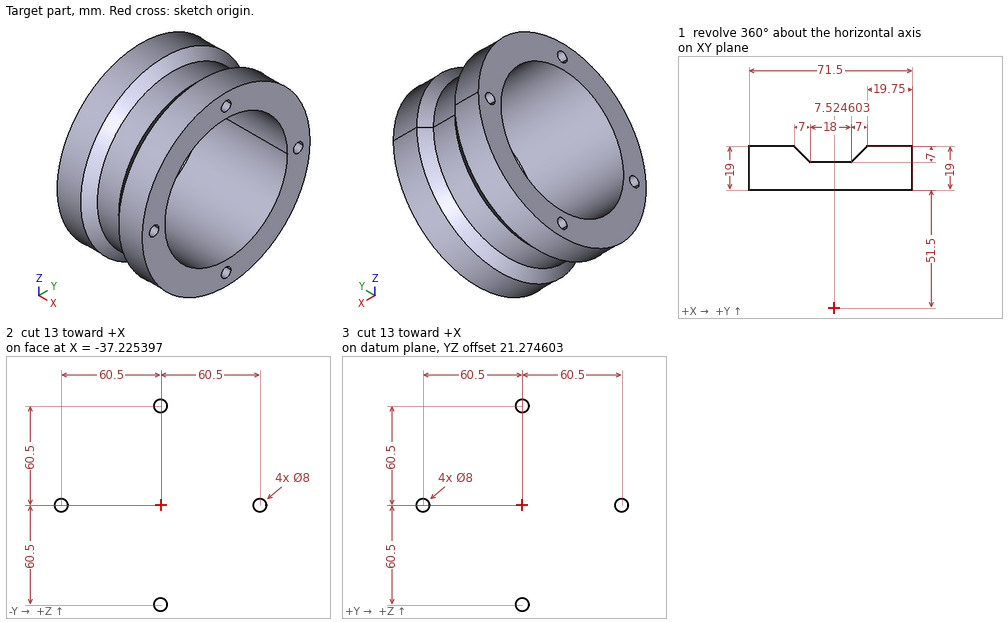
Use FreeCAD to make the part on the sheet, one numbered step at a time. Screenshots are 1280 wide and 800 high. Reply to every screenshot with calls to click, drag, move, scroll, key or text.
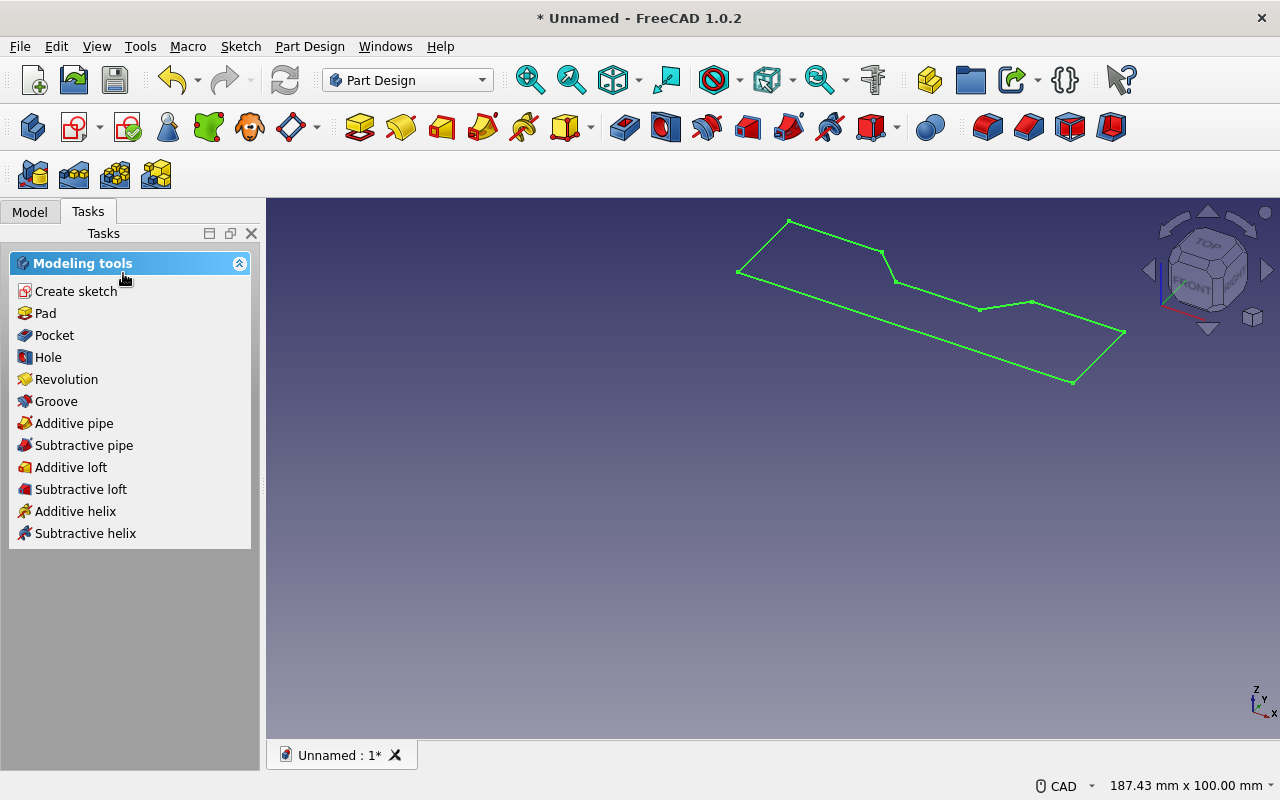
click(401, 128)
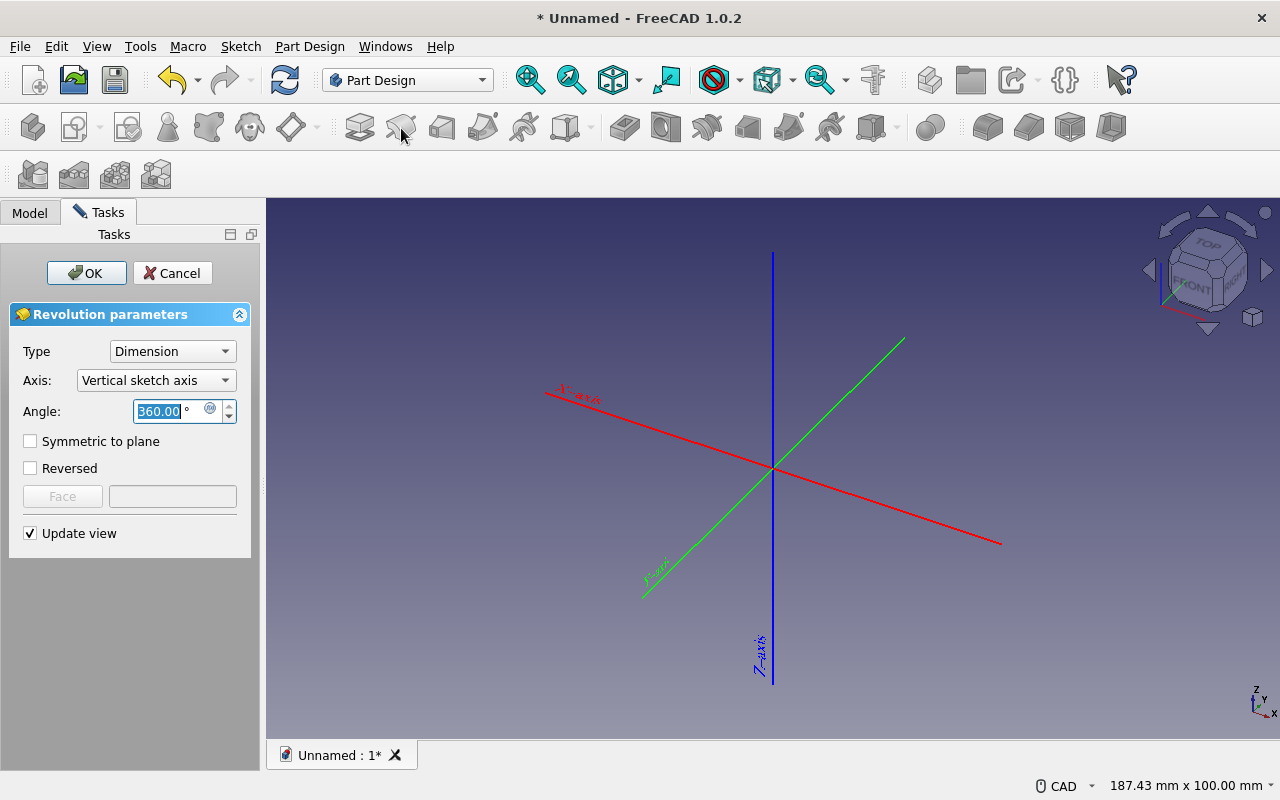
click(157, 380)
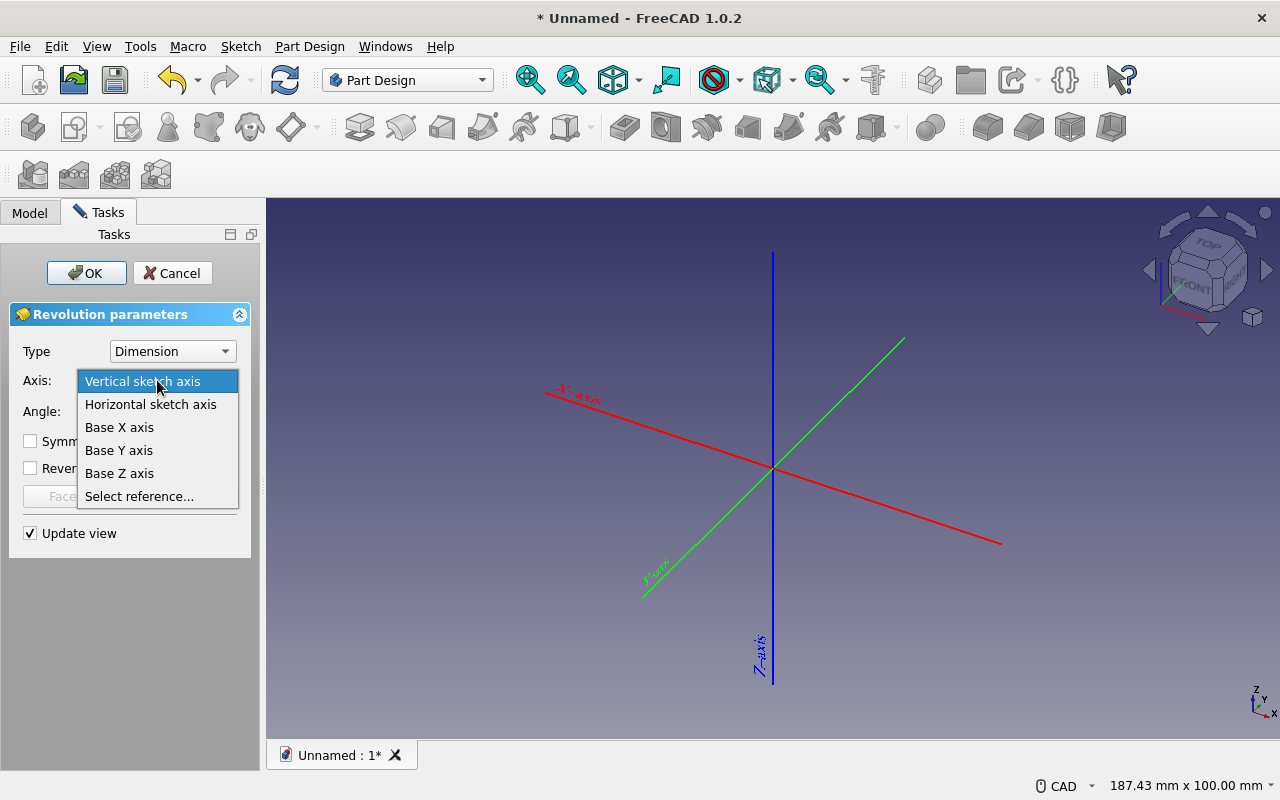
click(156, 404)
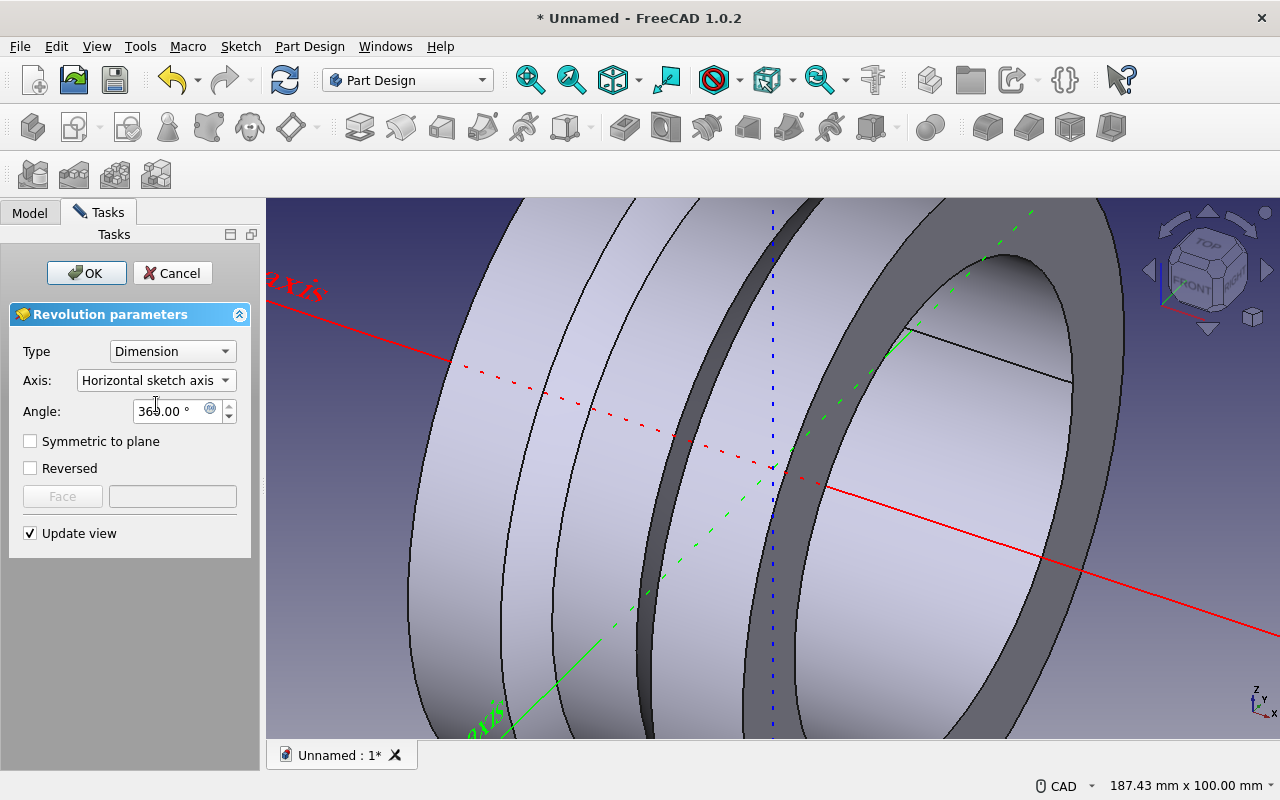
click(87, 273)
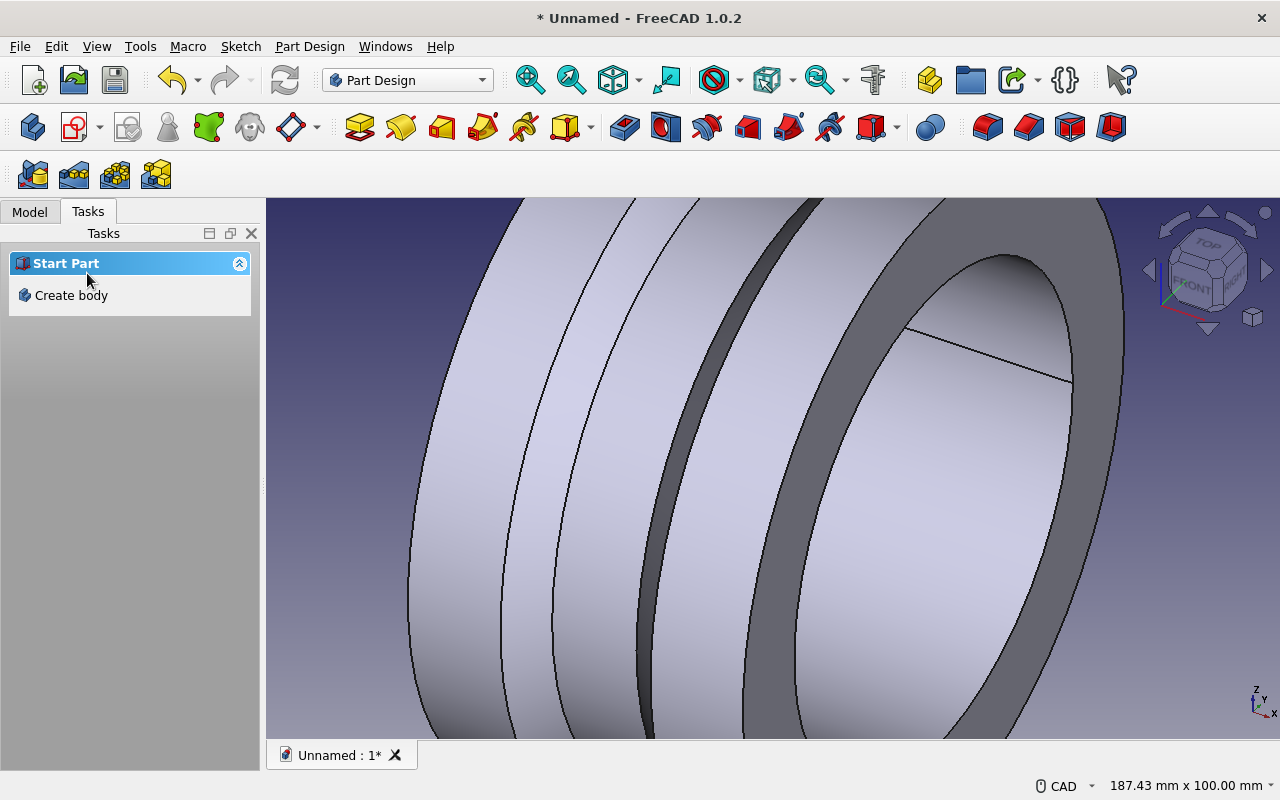
click(531, 80)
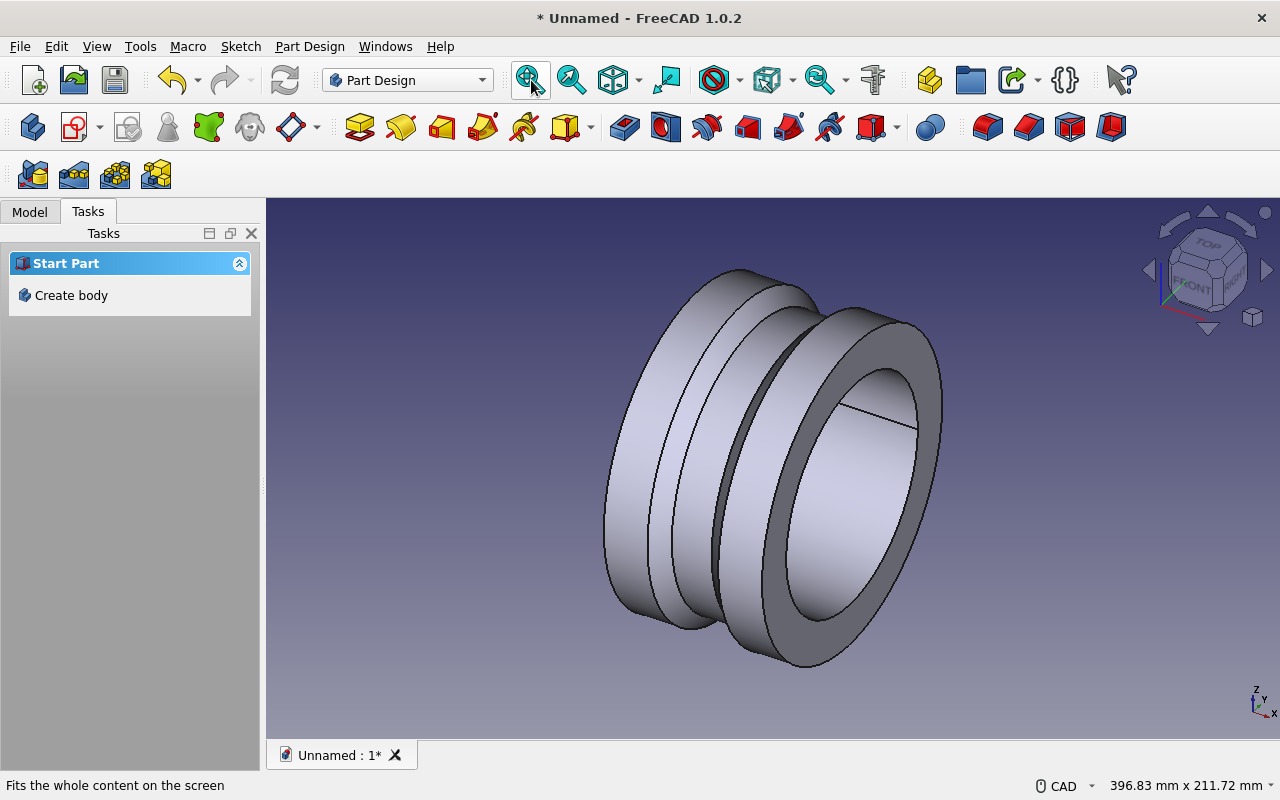
key(6)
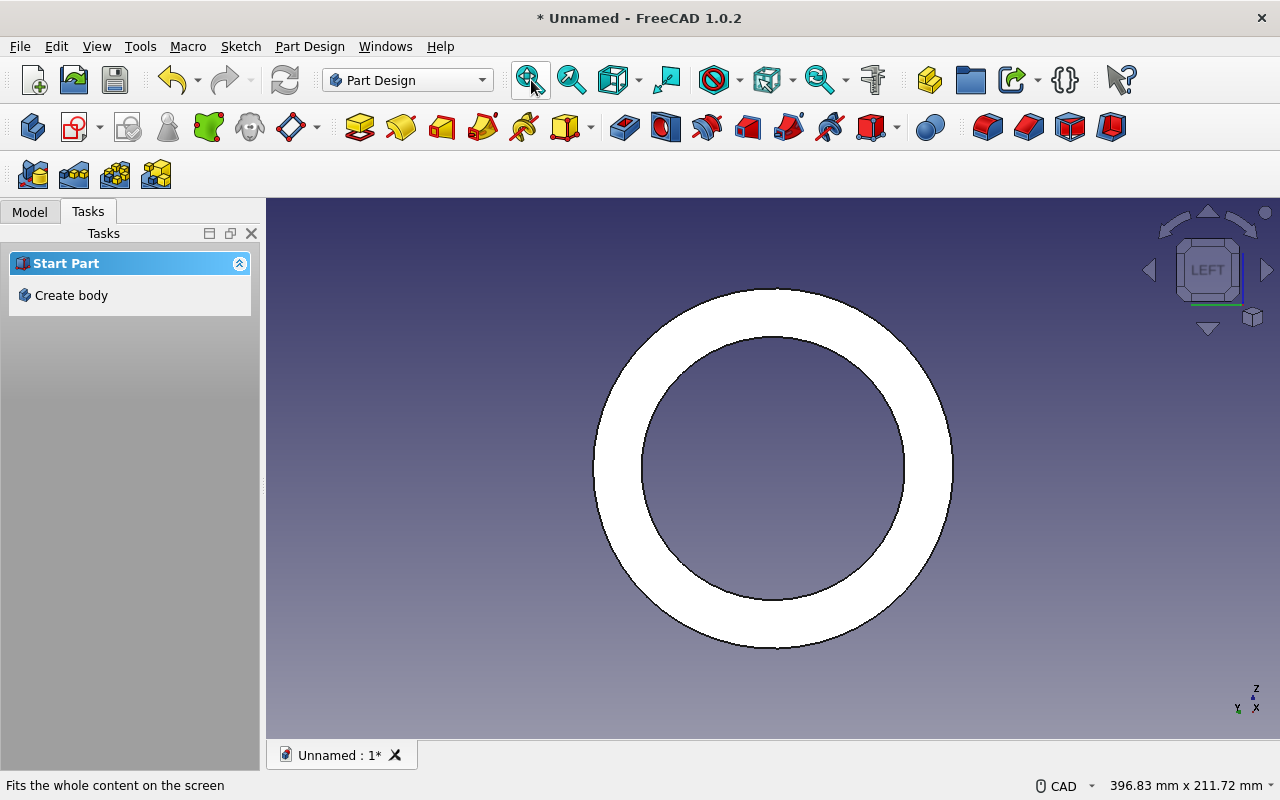
click(773, 622)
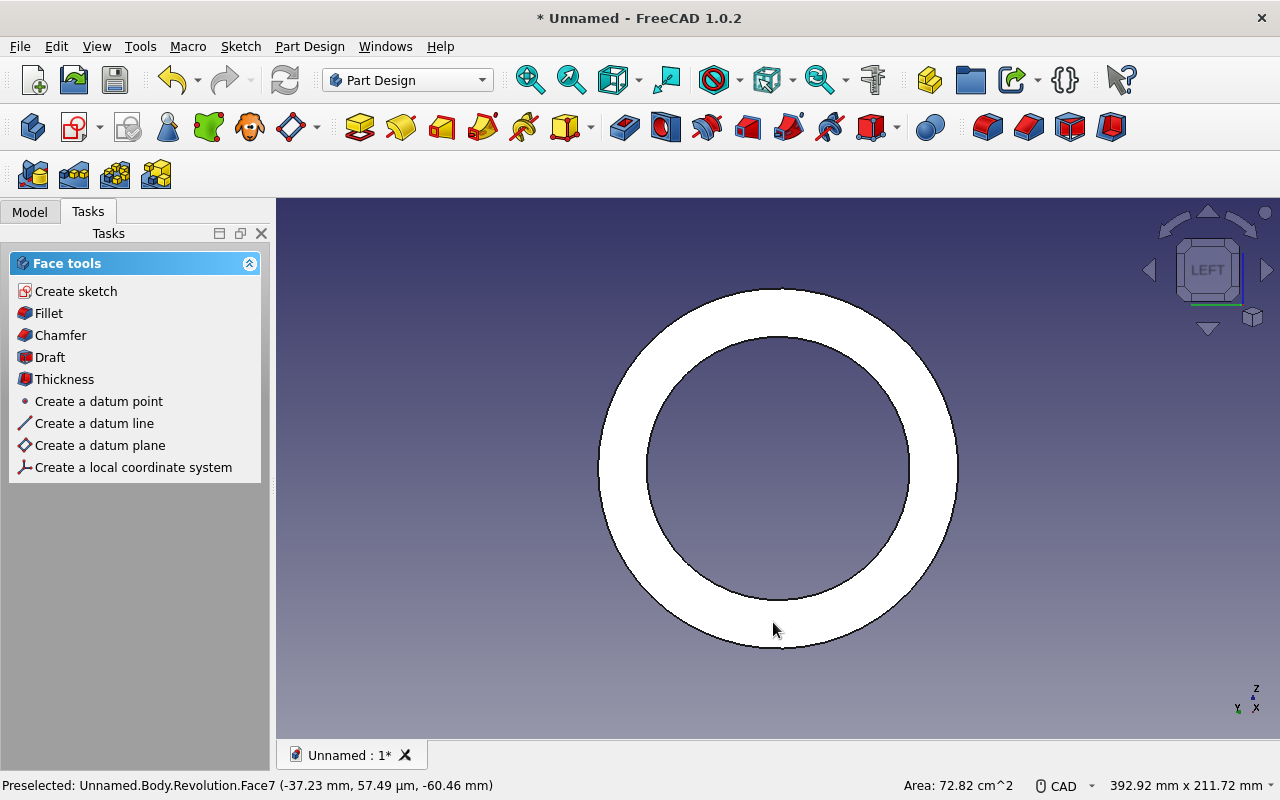
click(74, 128)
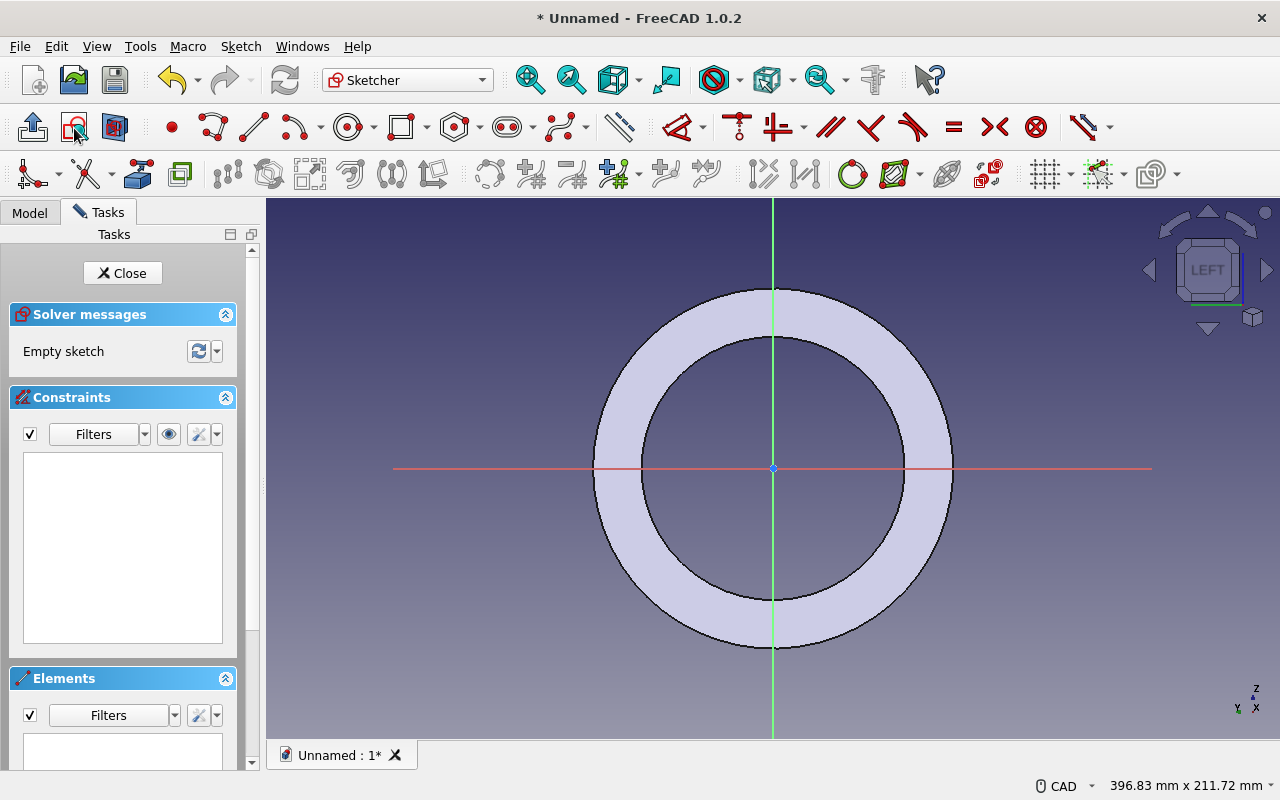
click(348, 128)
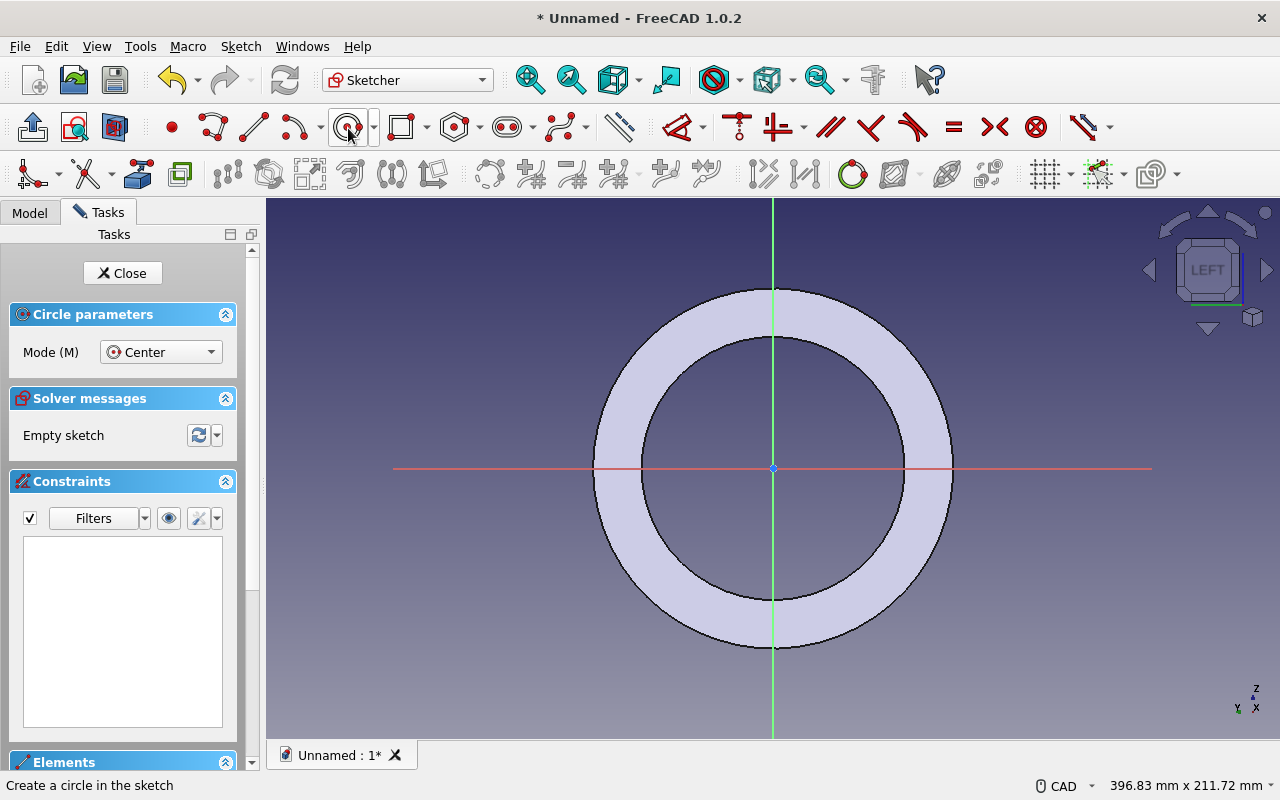
scroll(928, 468, up, 4)